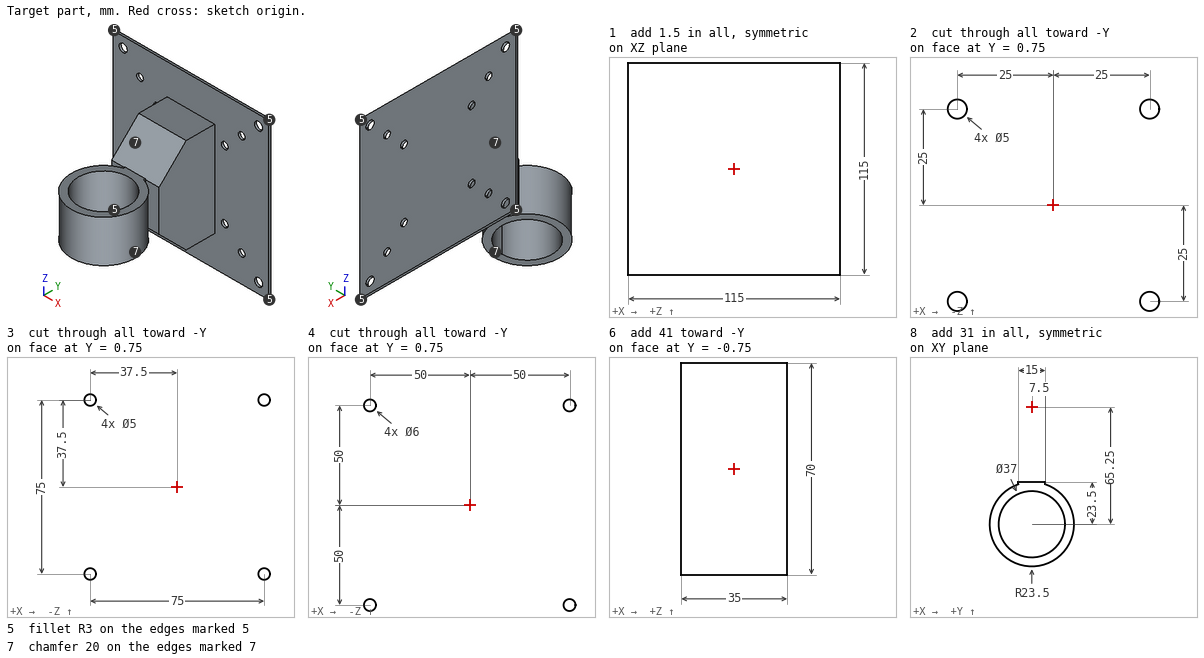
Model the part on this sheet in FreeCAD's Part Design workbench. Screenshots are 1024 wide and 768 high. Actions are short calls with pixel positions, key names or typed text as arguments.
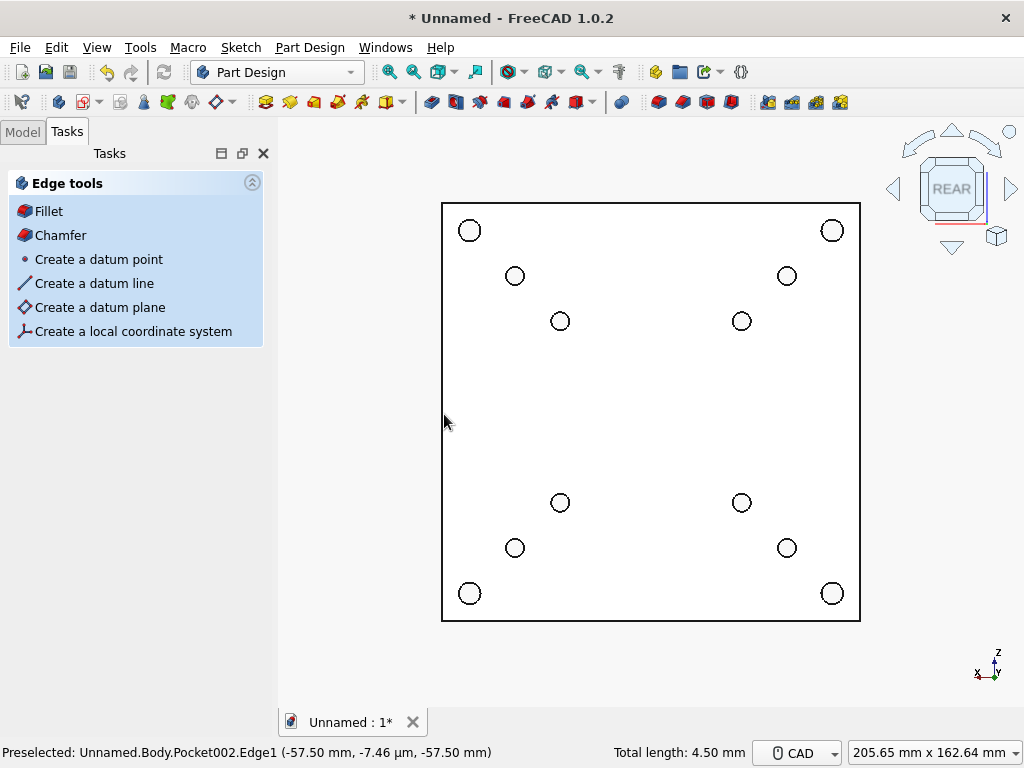
scroll(442, 202, up, 10)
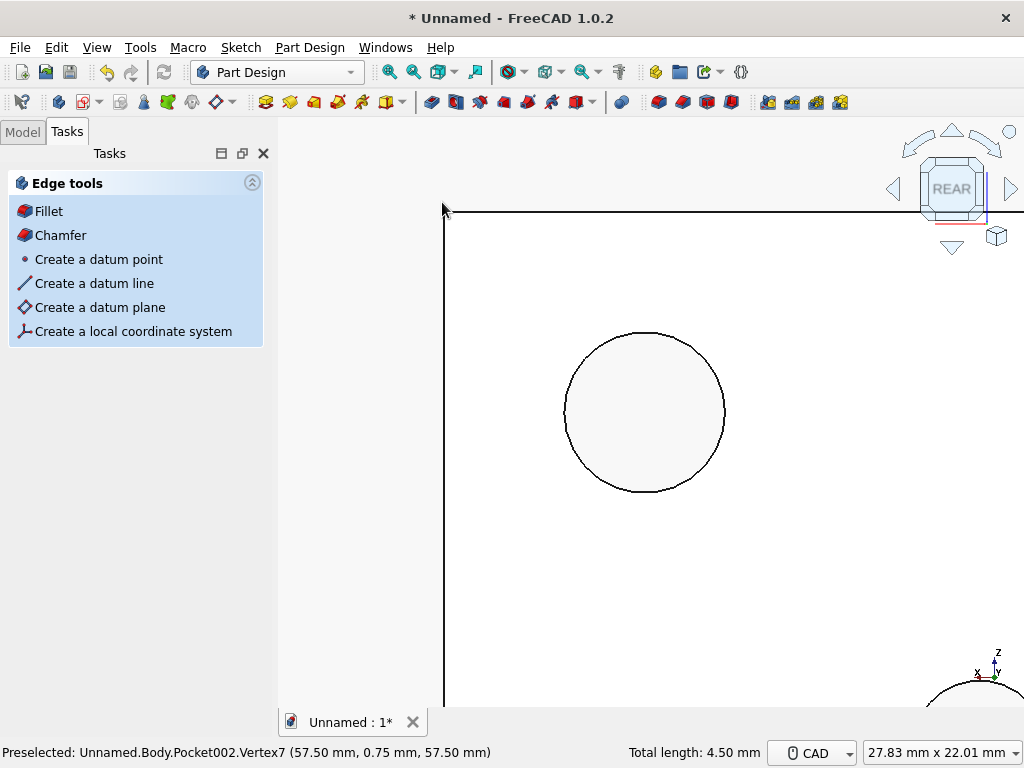
key(v)
key(f)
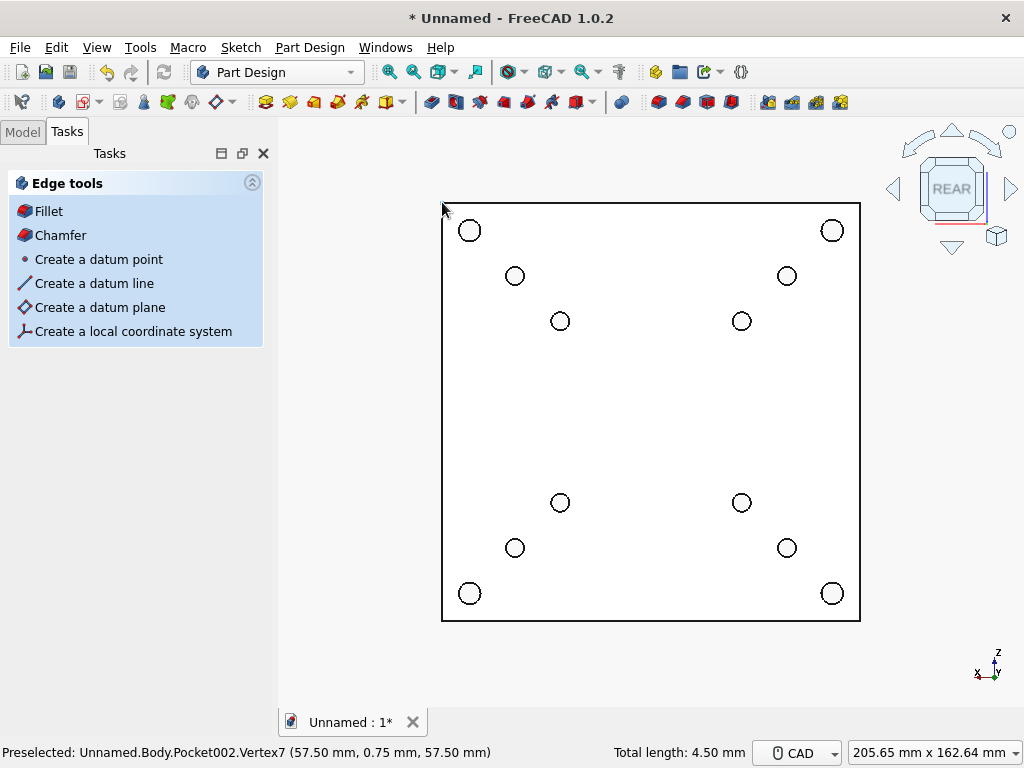
key(6)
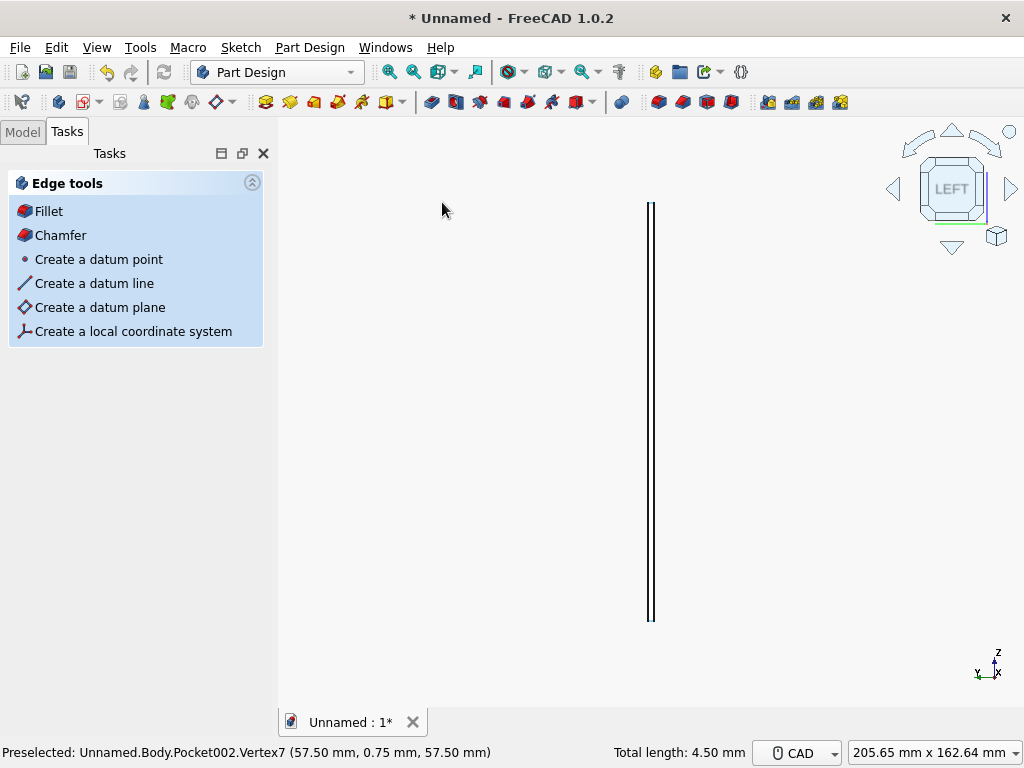
scroll(651, 202, up, 10)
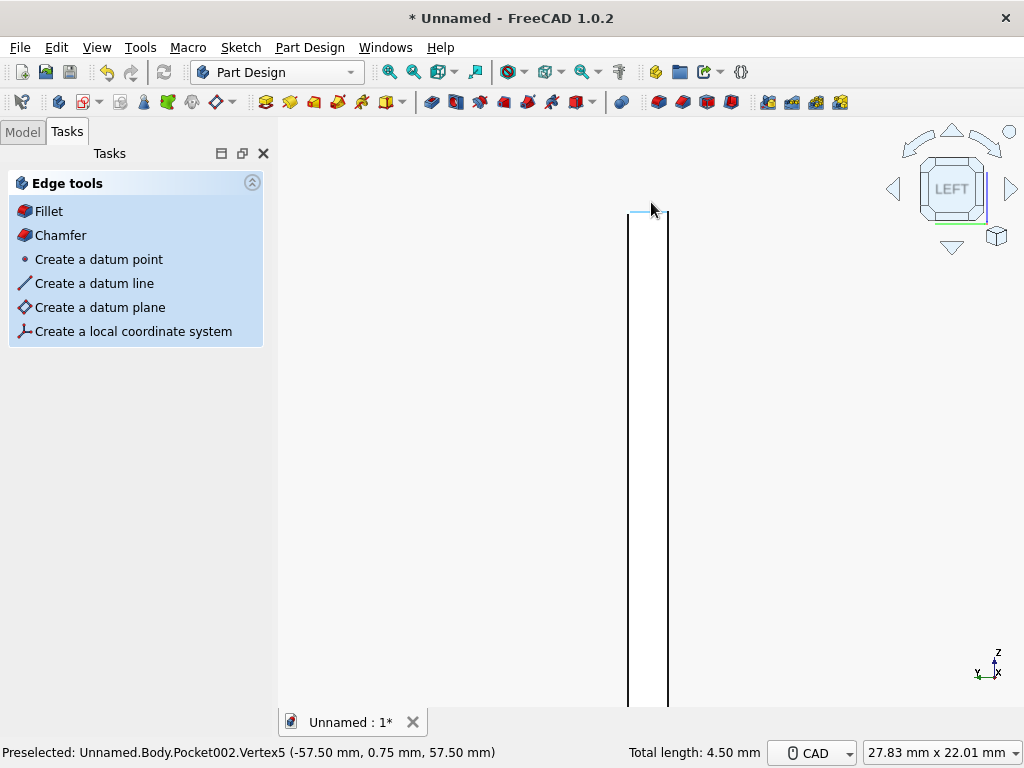
key(v)
key(f)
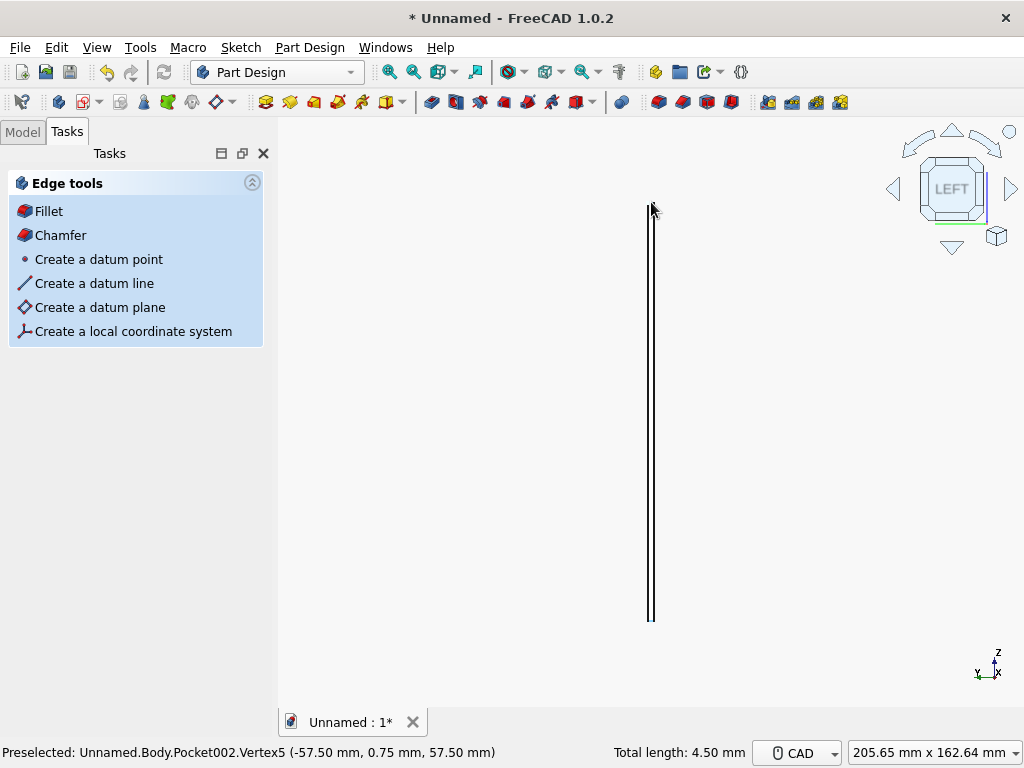
key(v)
key(3)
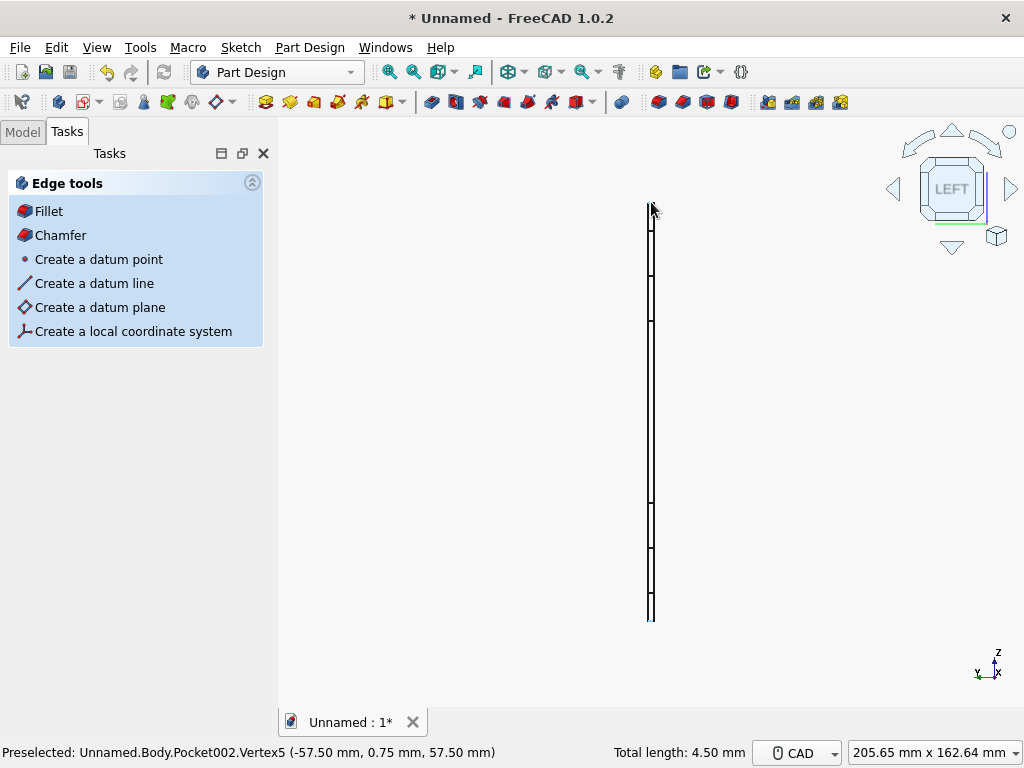
key(0)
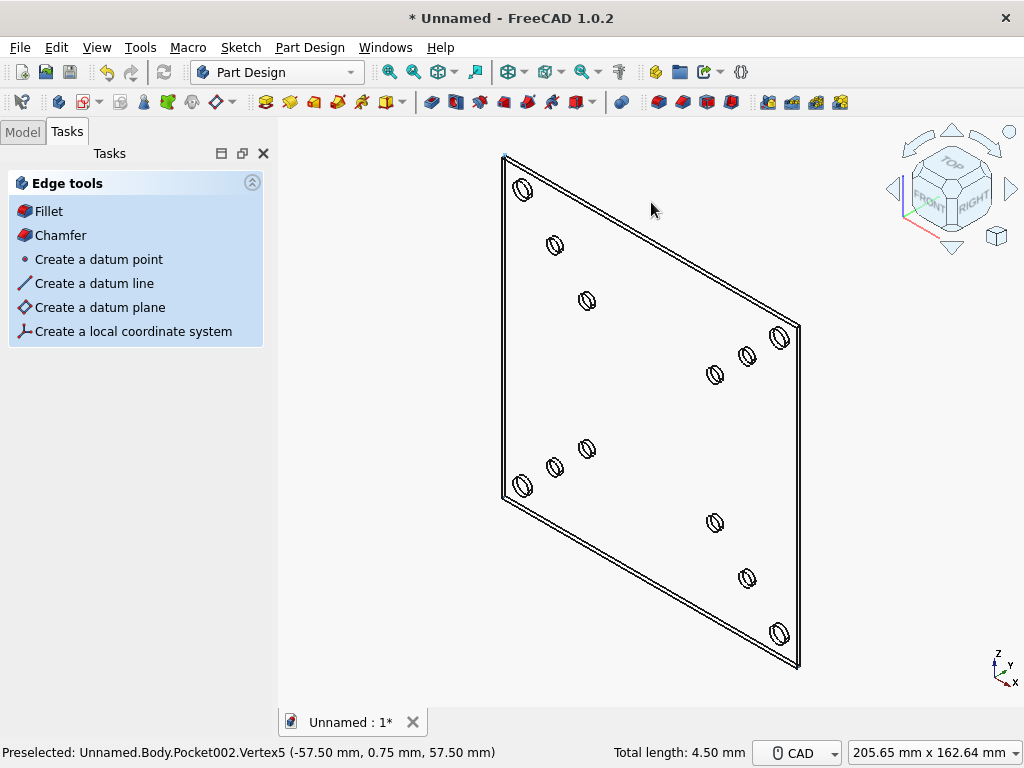
scroll(798, 326, up, 10)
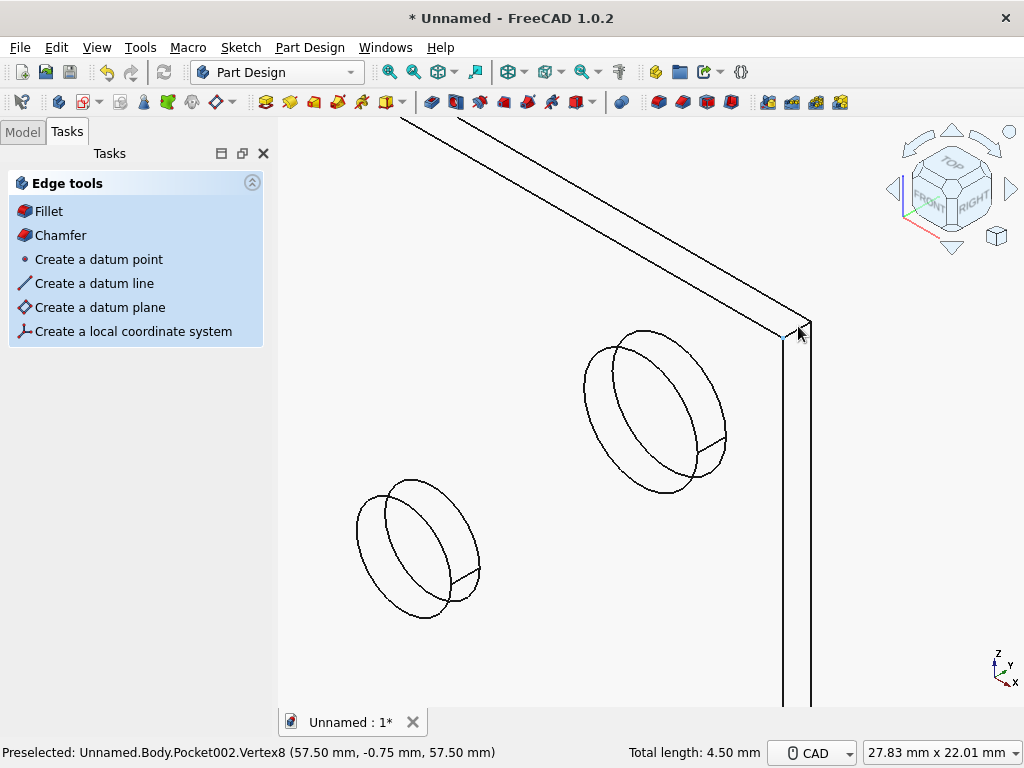
click(797, 329, ctrl)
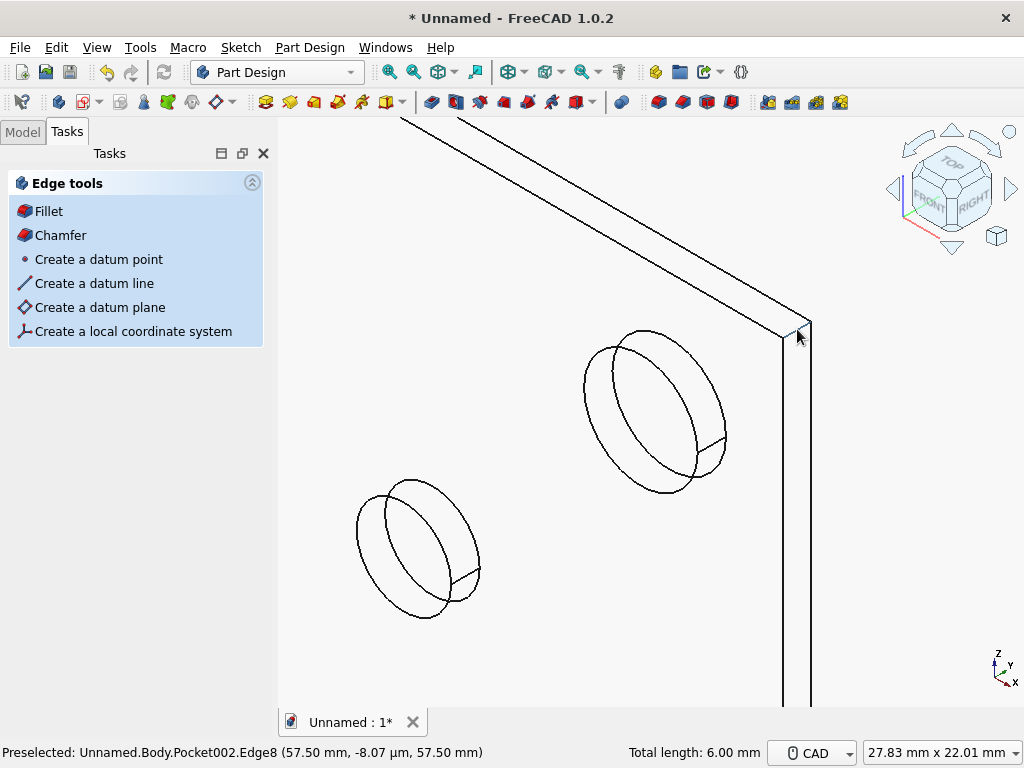
key(v)
key(1)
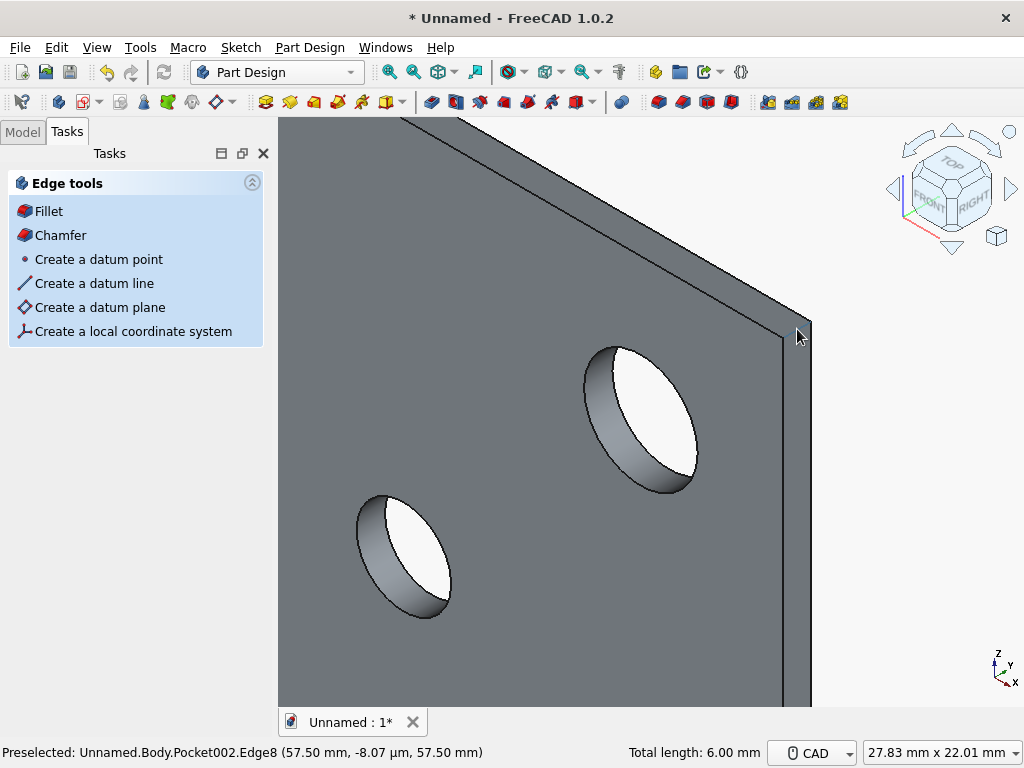
click(660, 102)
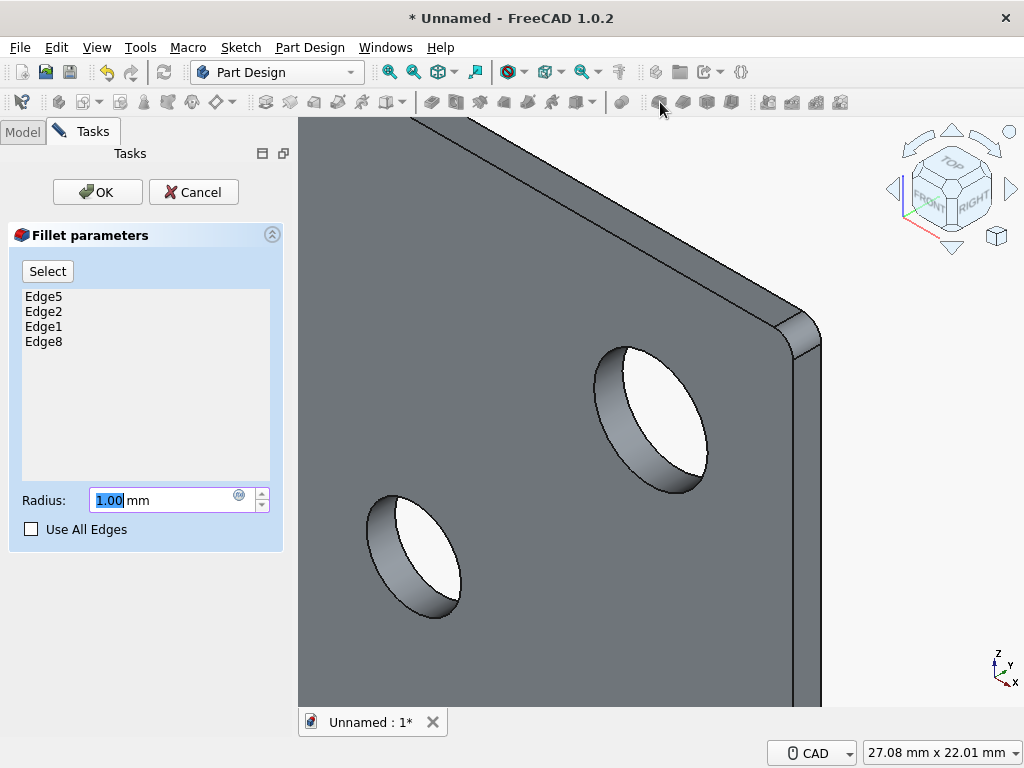
text(3)
key(Tab)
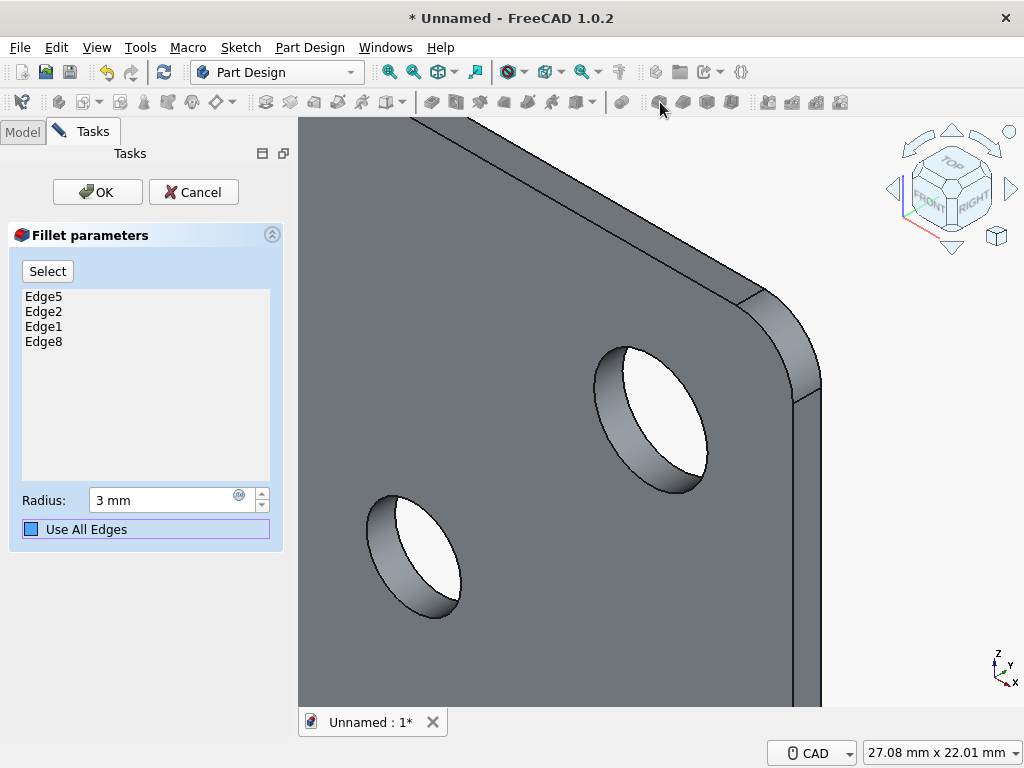
click(98, 192)